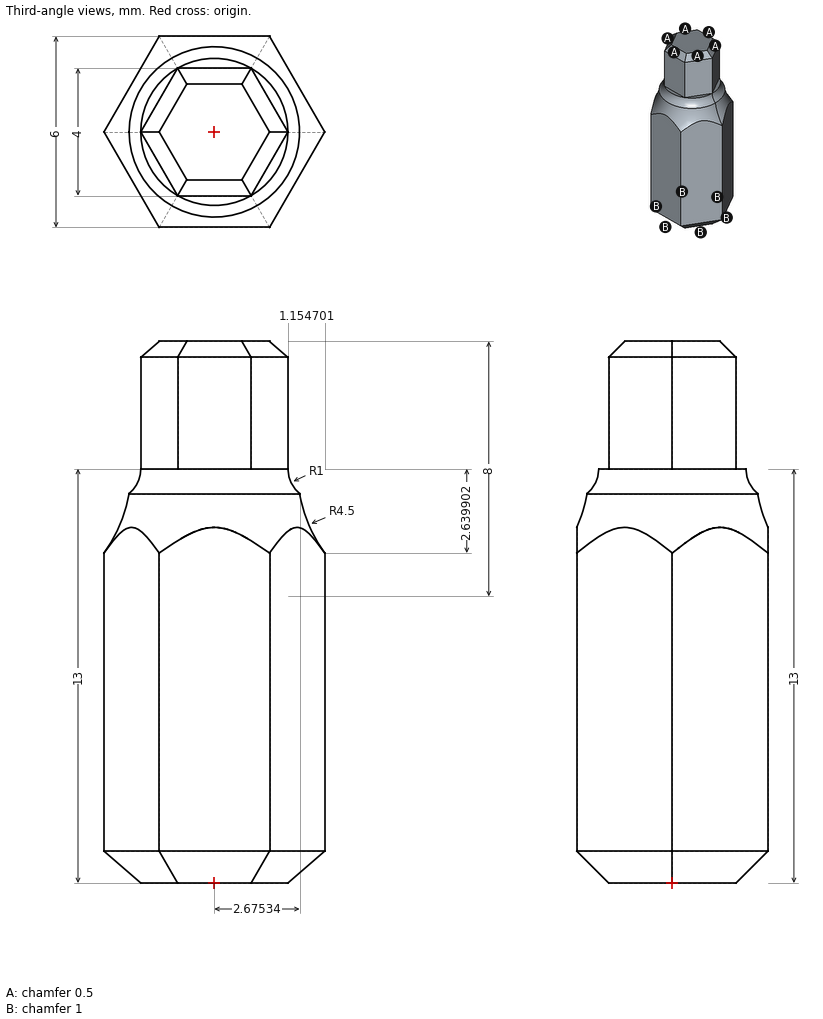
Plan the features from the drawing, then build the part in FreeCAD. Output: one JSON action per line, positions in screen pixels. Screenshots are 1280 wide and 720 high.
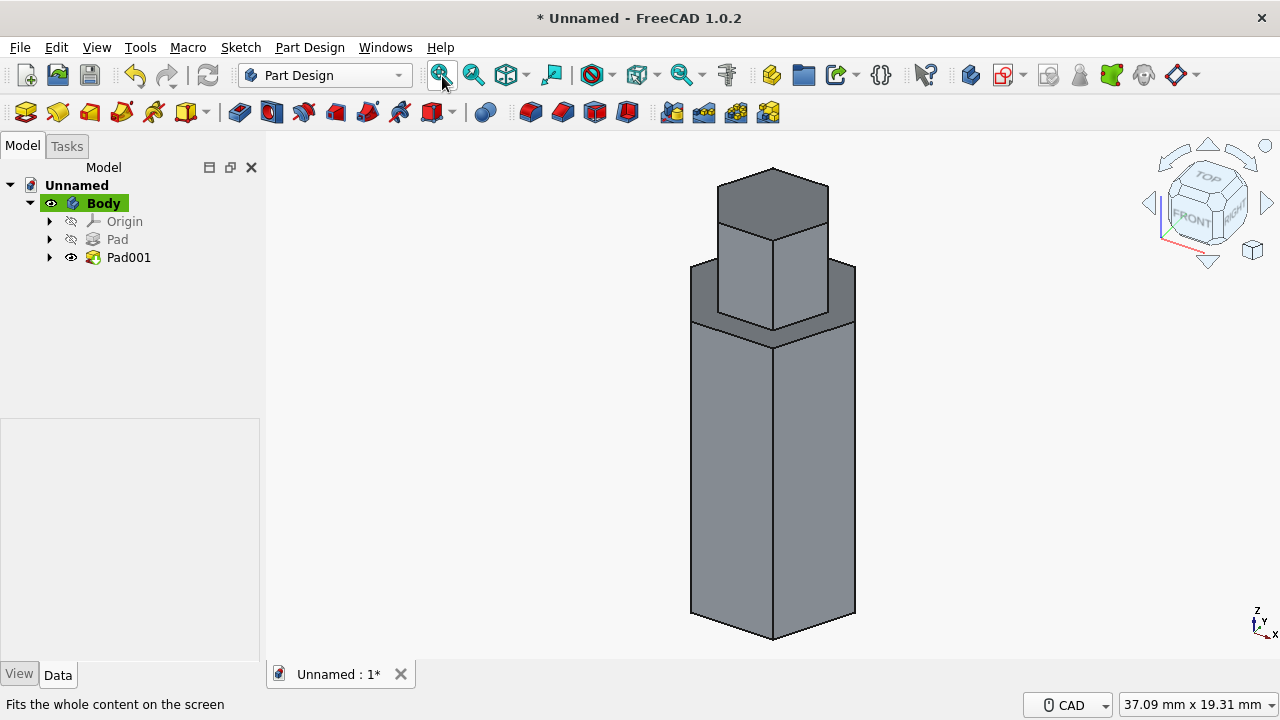
{"action": "left_click", "coordinate": [1004, 76]}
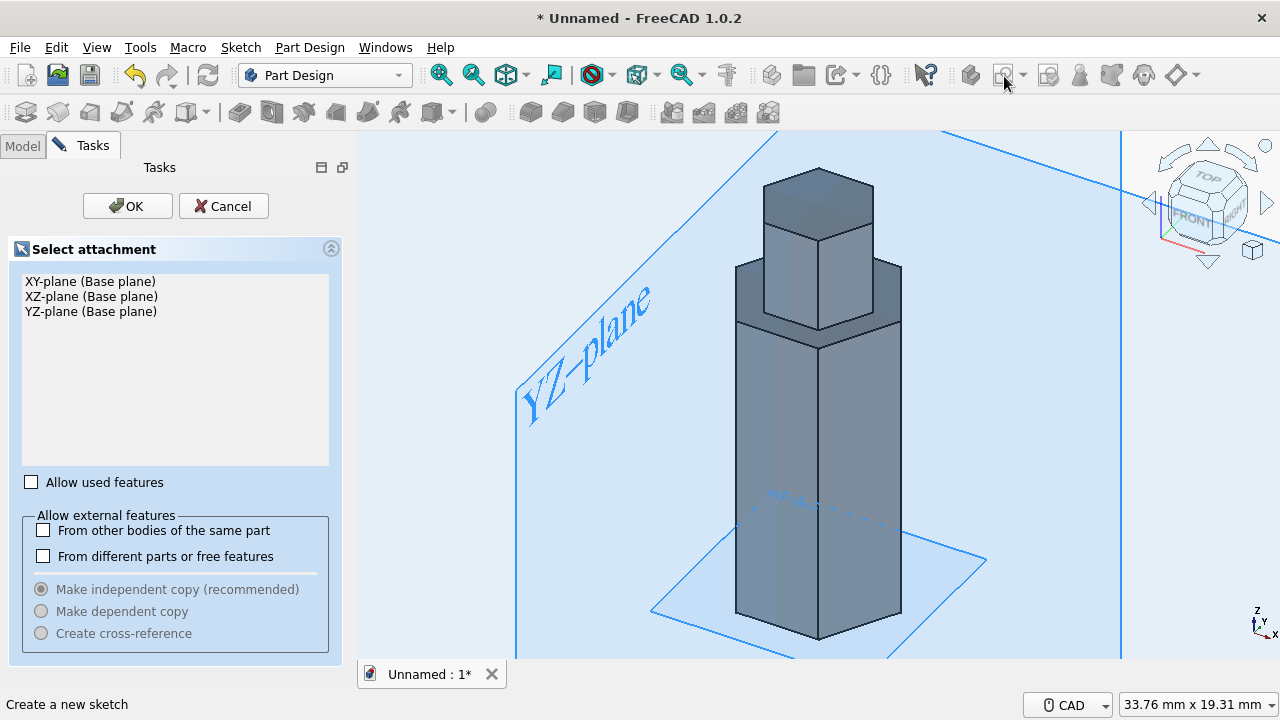
{"action": "left_click", "coordinate": [82, 296]}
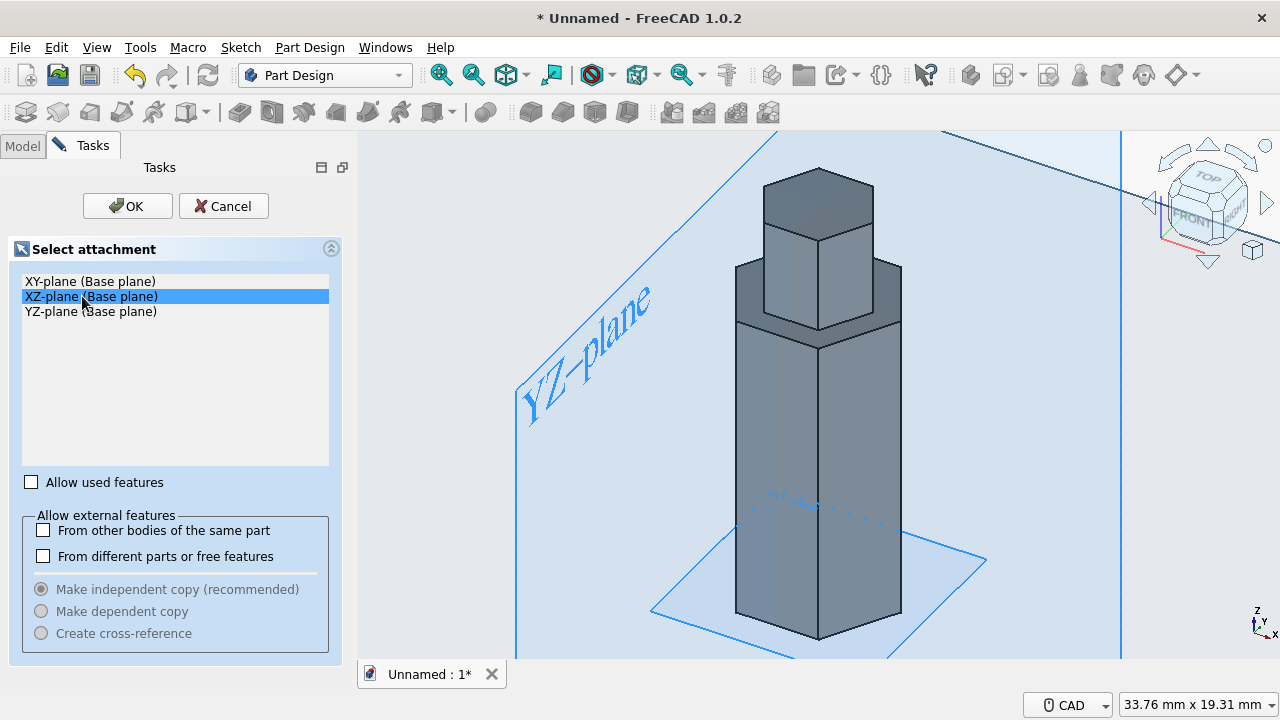
{"action": "left_click", "coordinate": [128, 206]}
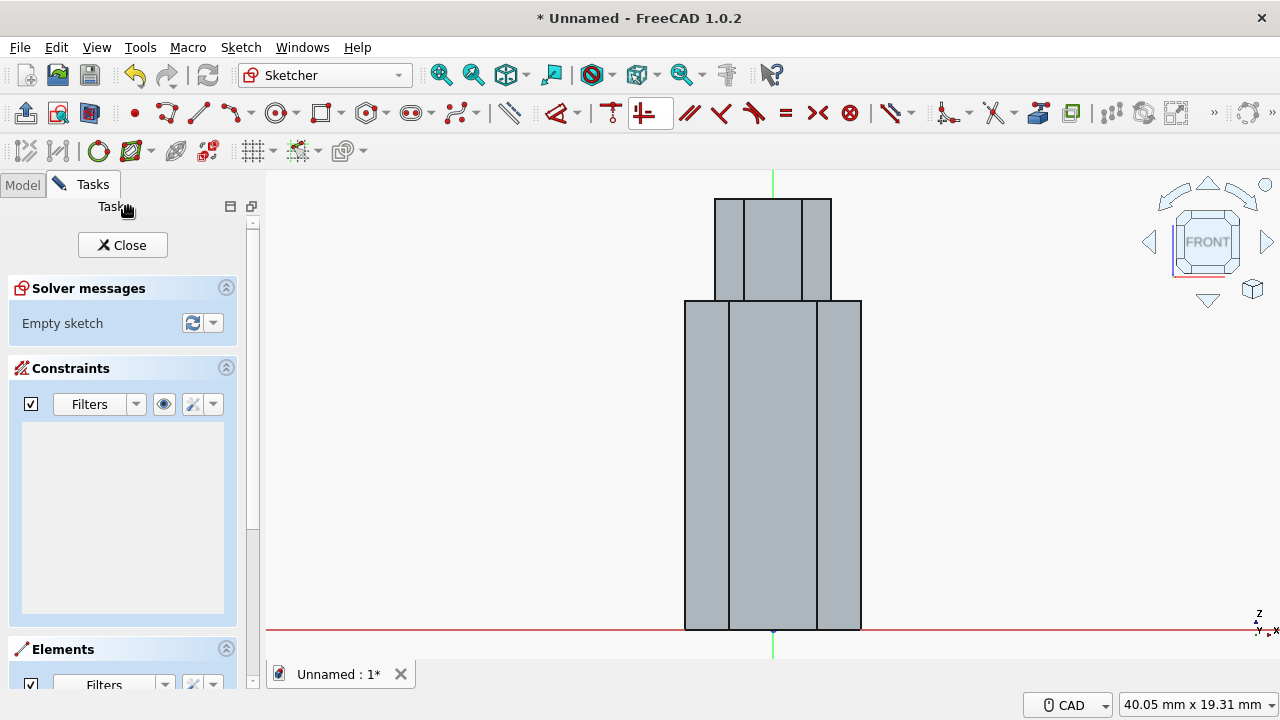
{"action": "left_click", "coordinate": [90, 114]}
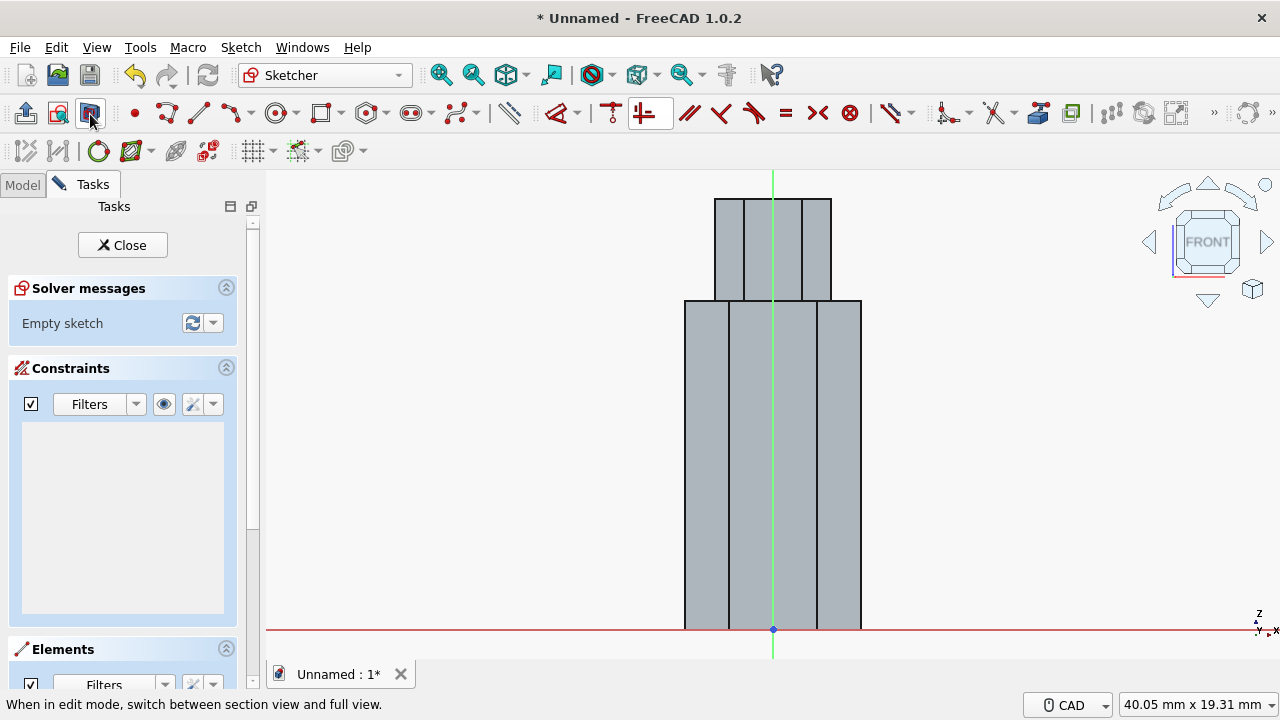
{"action": "scroll", "coordinate": [882, 314], "scroll_direction": "up", "scroll_amount": 8}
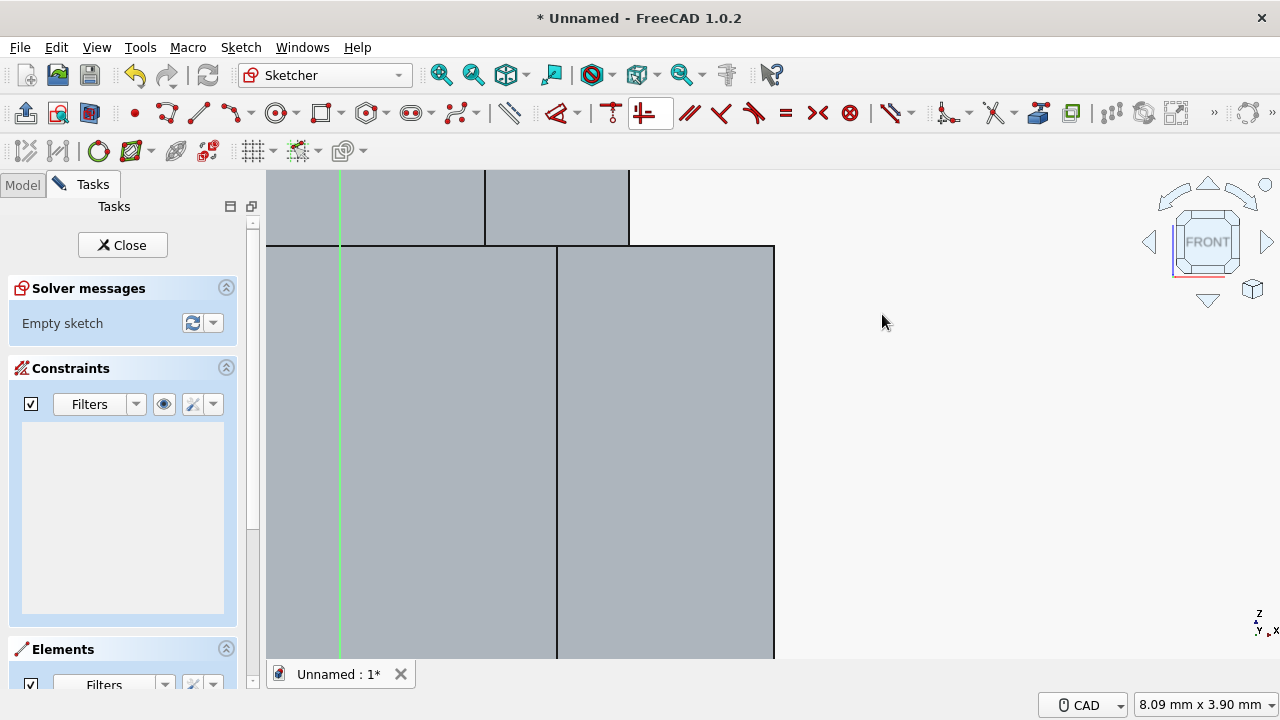
{"action": "left_click", "coordinate": [168, 114]}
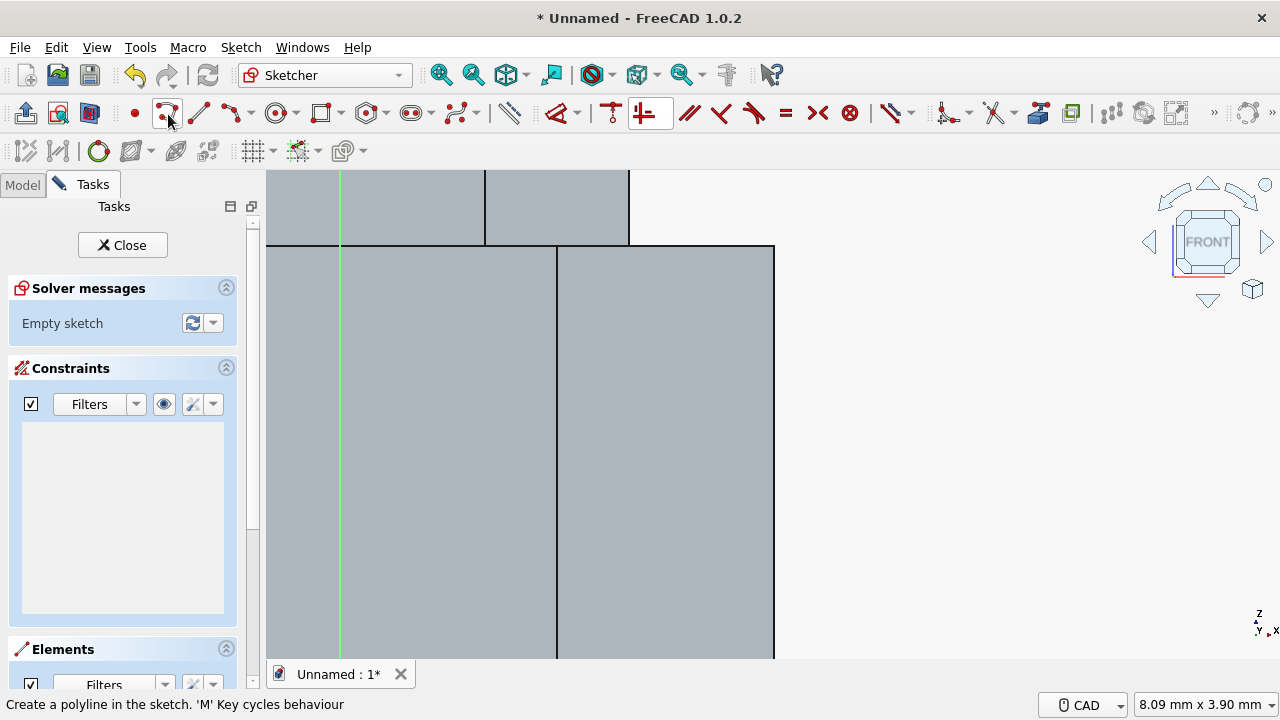
{"action": "left_click", "coordinate": [629, 246]}
{"action": "left_click", "coordinate": [774, 246]}
{"action": "left_click", "coordinate": [774, 577]}
{"action": "right_click", "coordinate": [774, 577]}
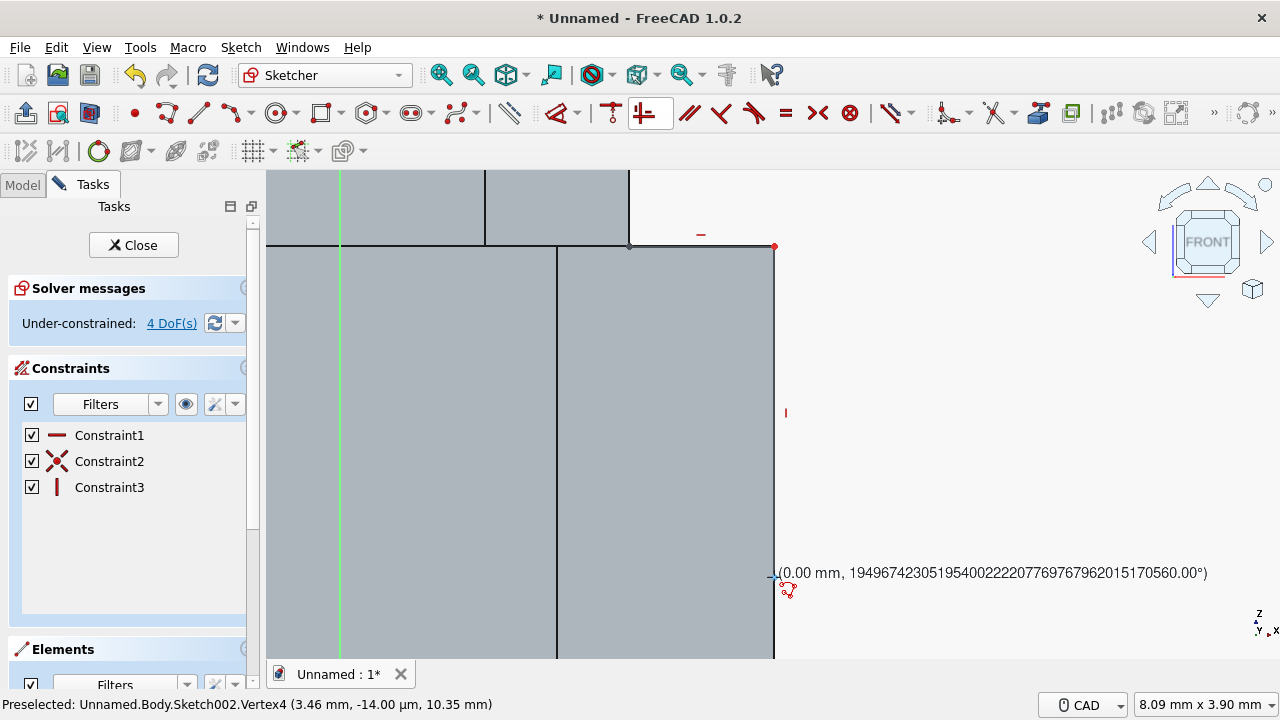
{"action": "left_click", "coordinate": [232, 114]}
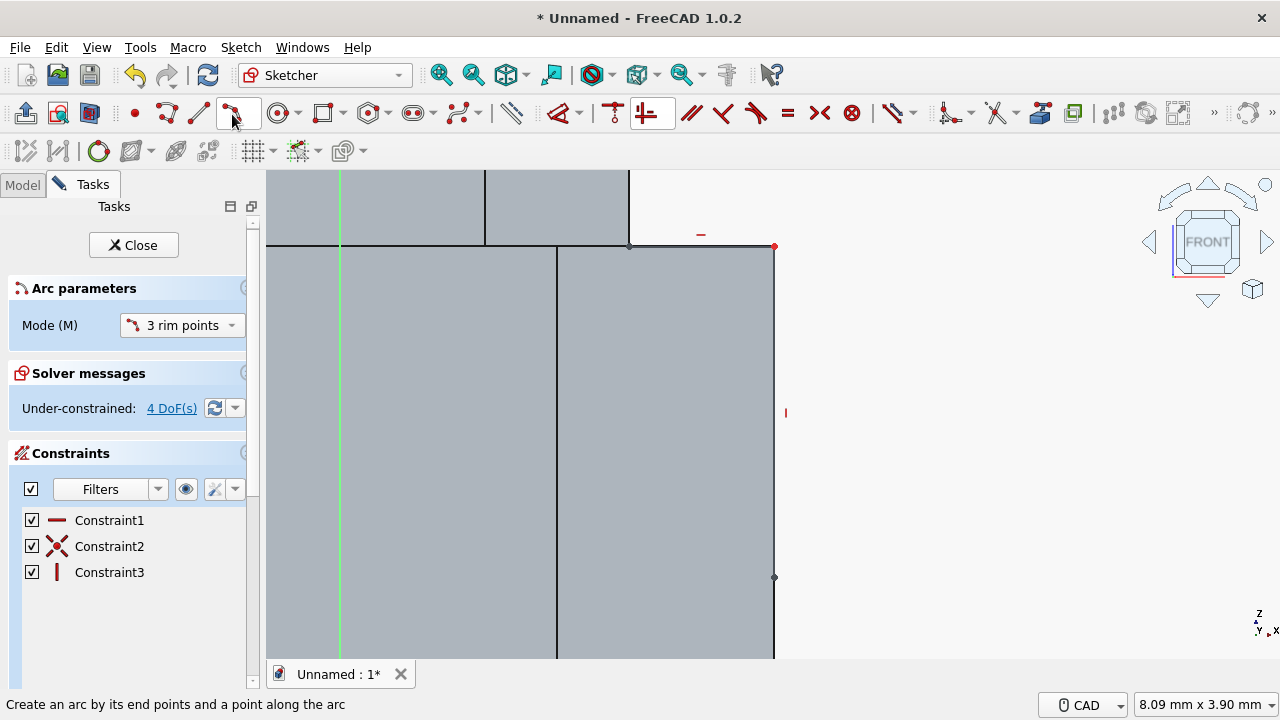
{"action": "left_click", "coordinate": [774, 578]}
{"action": "left_click", "coordinate": [675, 343]}
{"action": "left_click", "coordinate": [711, 466]}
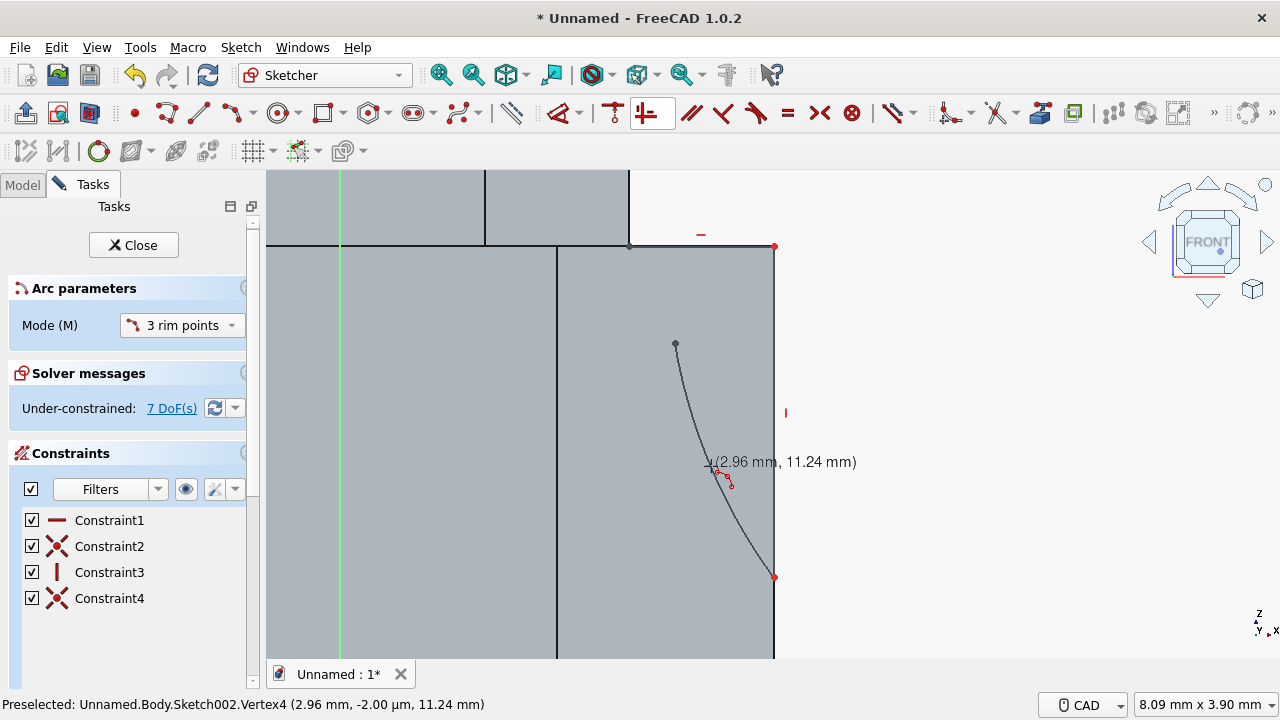
{"action": "left_click", "coordinate": [675, 344]}
{"action": "left_click", "coordinate": [629, 247]}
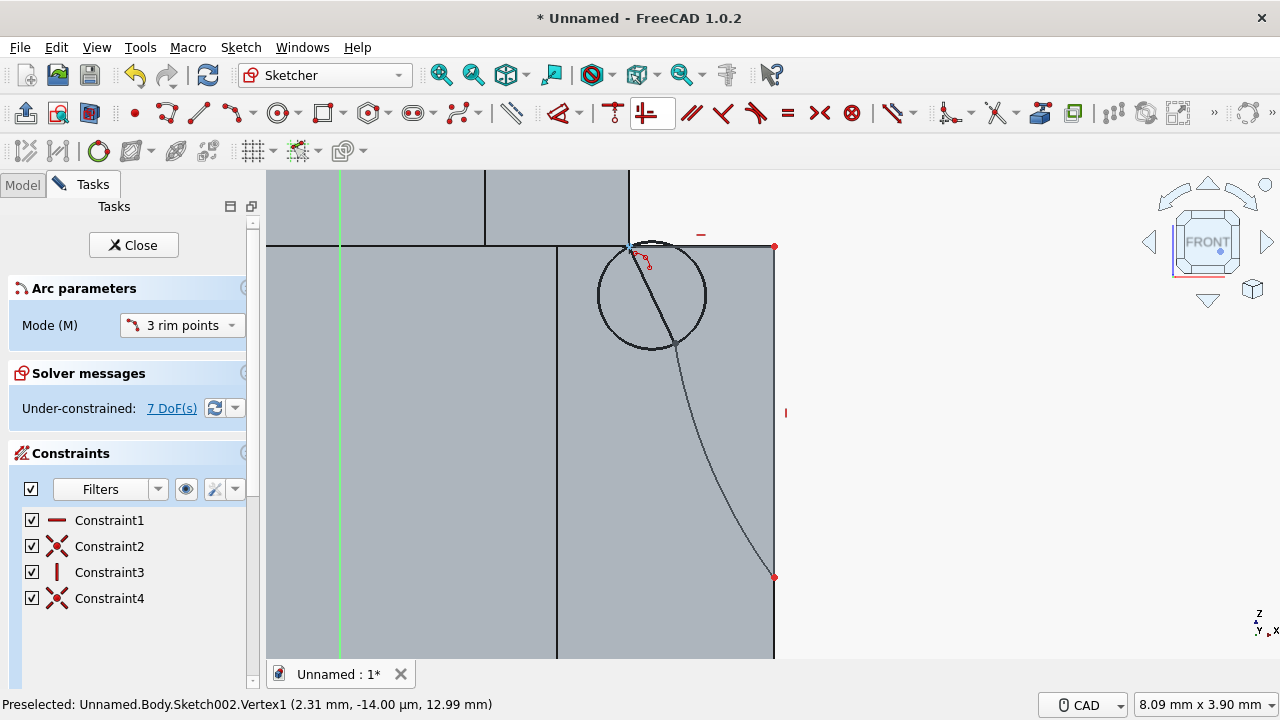
{"action": "scroll", "coordinate": [641, 300], "scroll_direction": "up", "scroll_amount": 2}